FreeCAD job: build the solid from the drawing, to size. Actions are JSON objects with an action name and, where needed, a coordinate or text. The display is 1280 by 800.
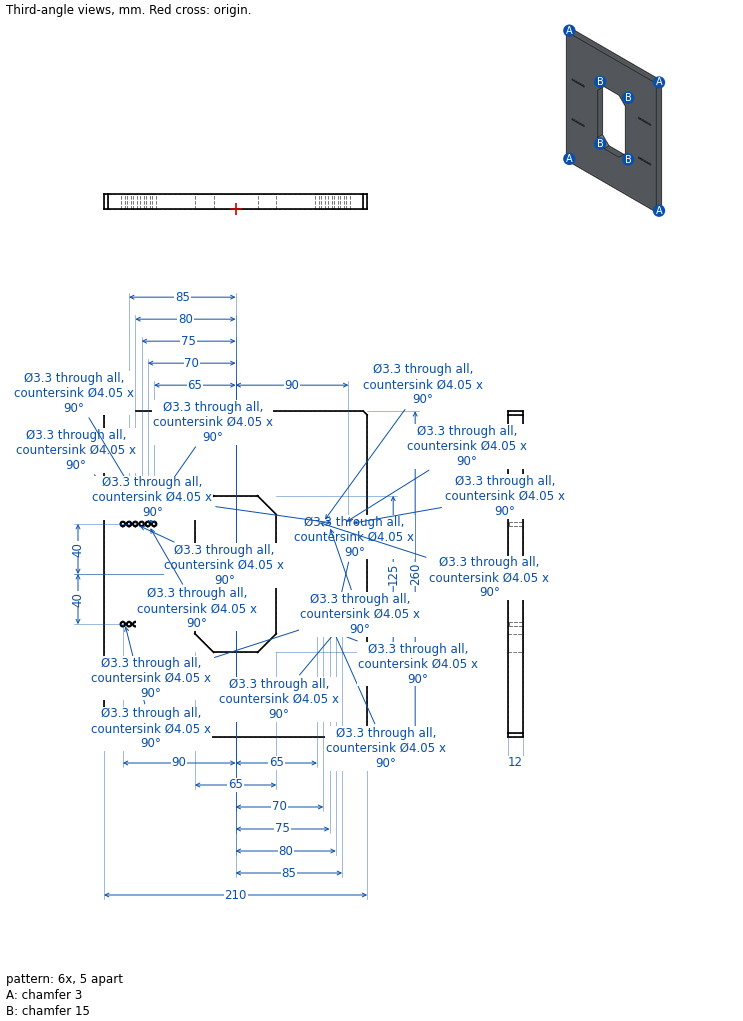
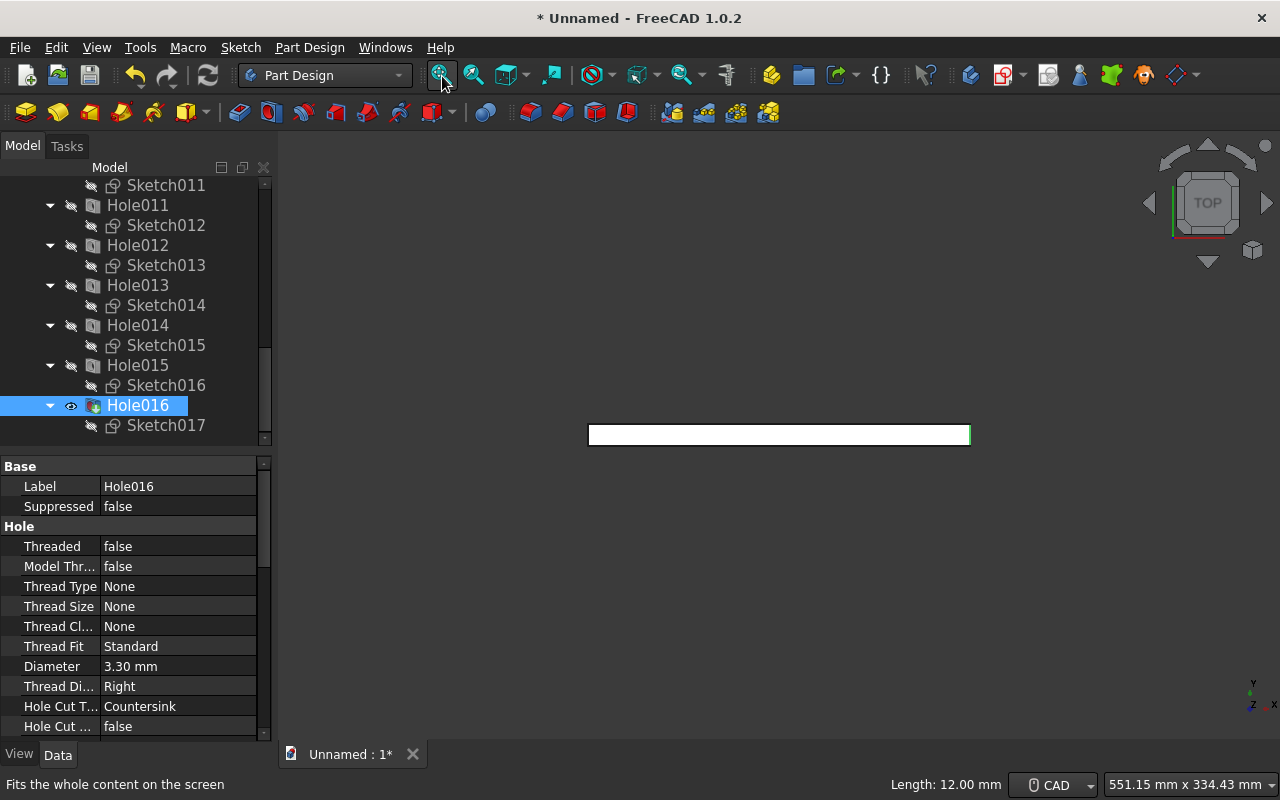
{"action": "left_click", "coordinate": [442, 76]}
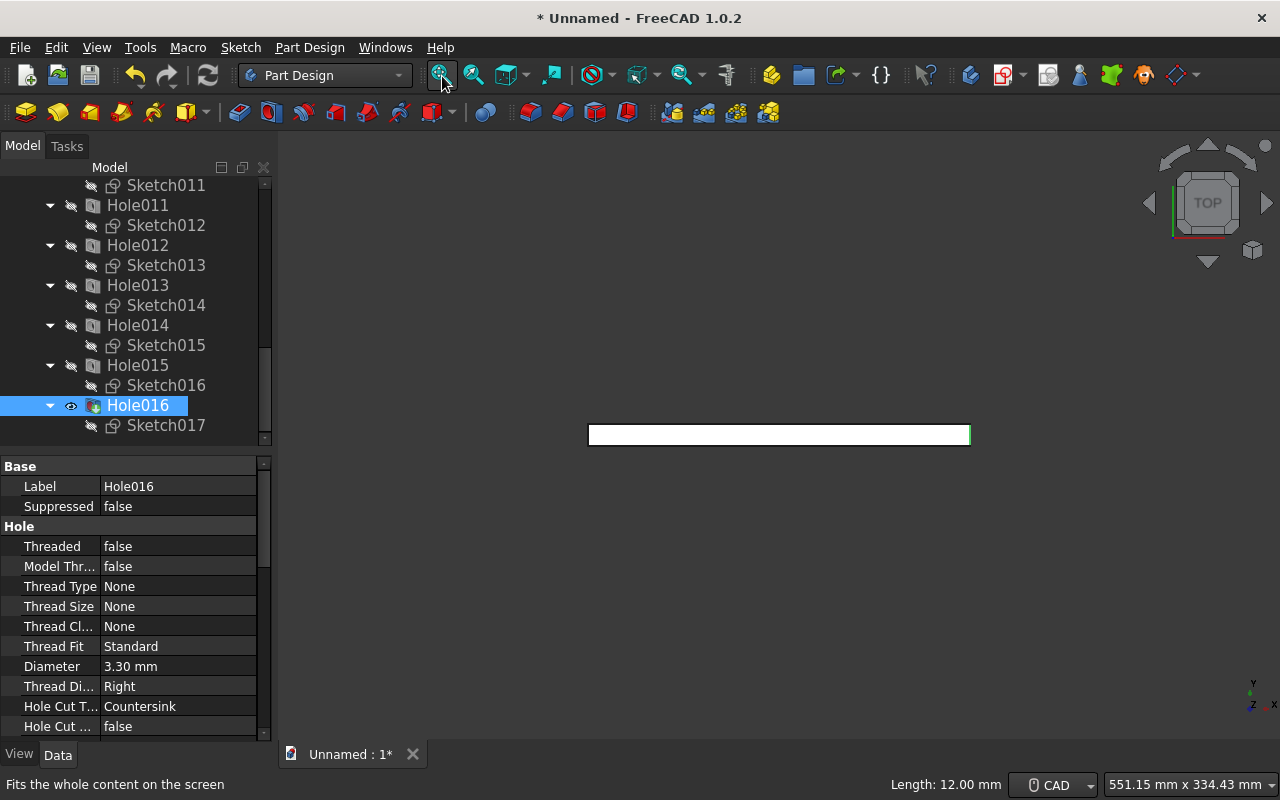
{"action": "left_click", "coordinate": [588, 434], "text": "ctrl"}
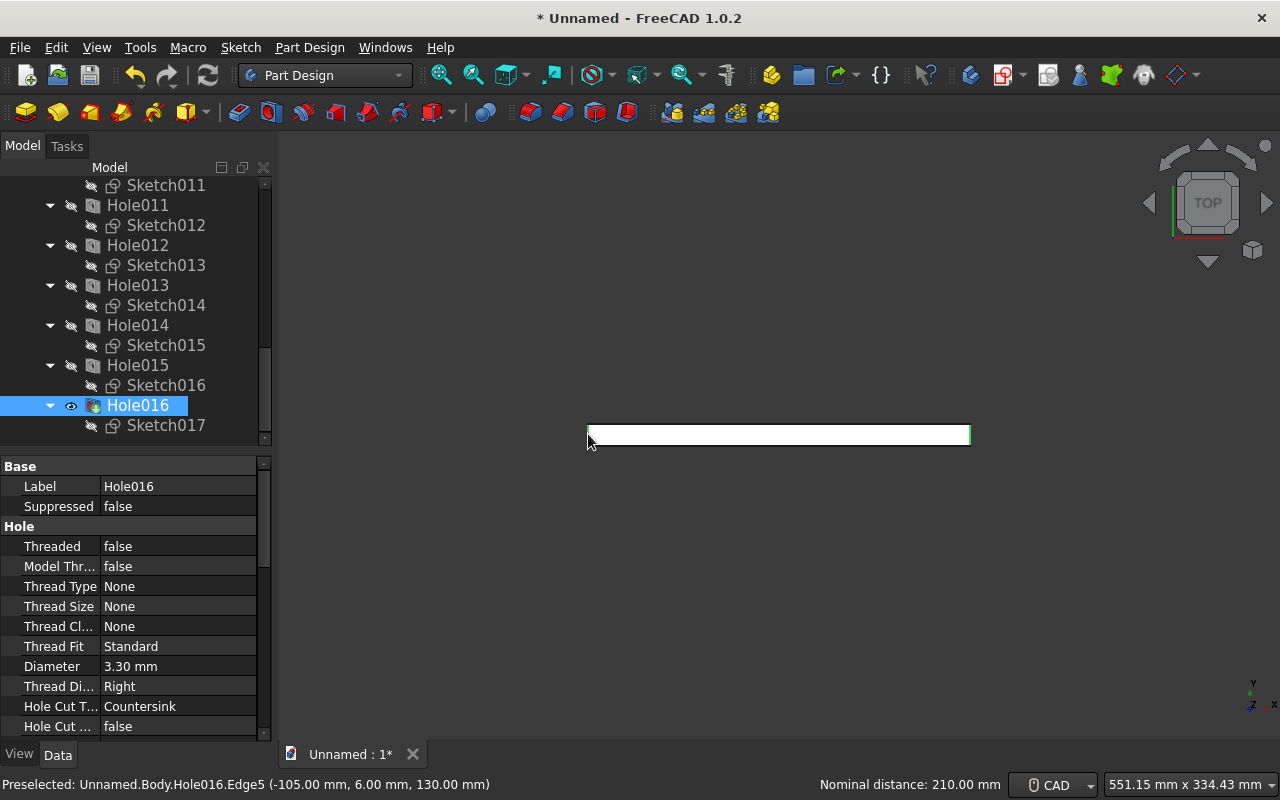
{"action": "scroll", "coordinate": [588, 434], "scroll_direction": "up", "scroll_amount": 4}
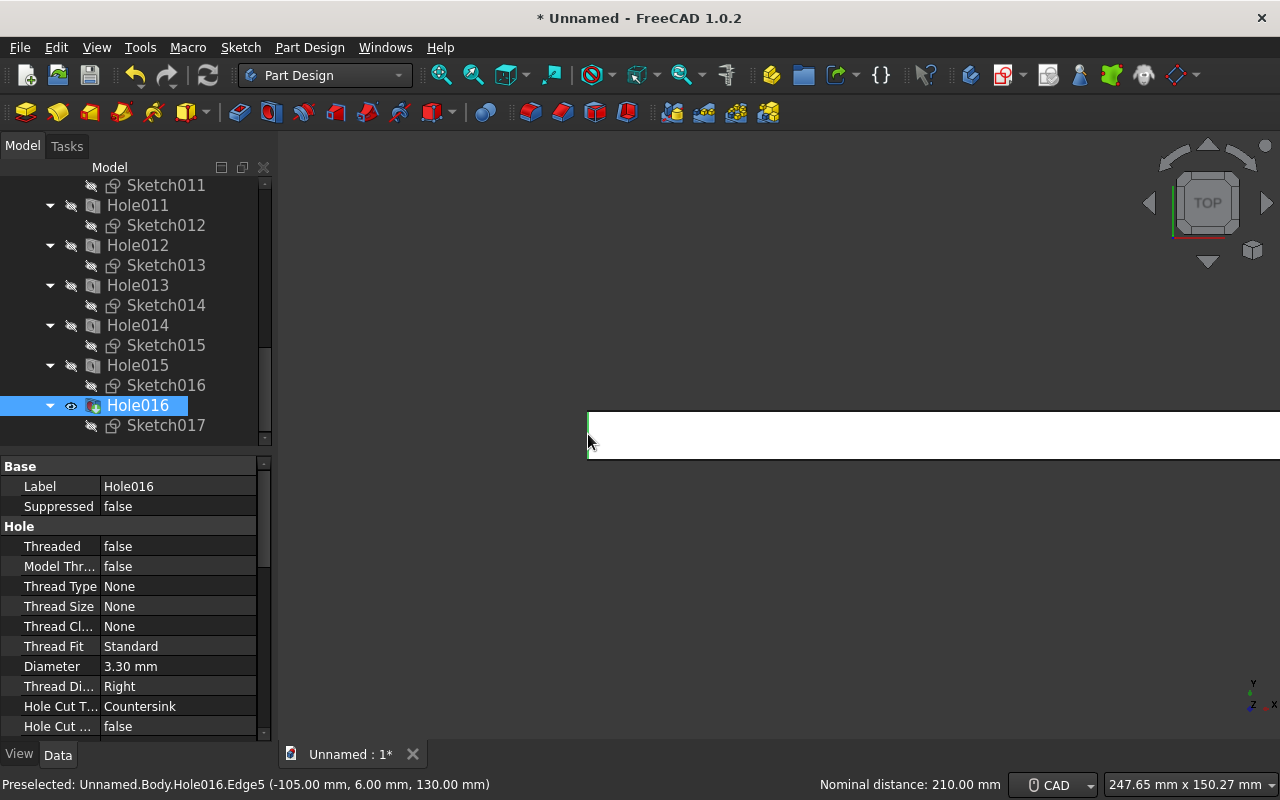
{"action": "left_click", "coordinate": [442, 76]}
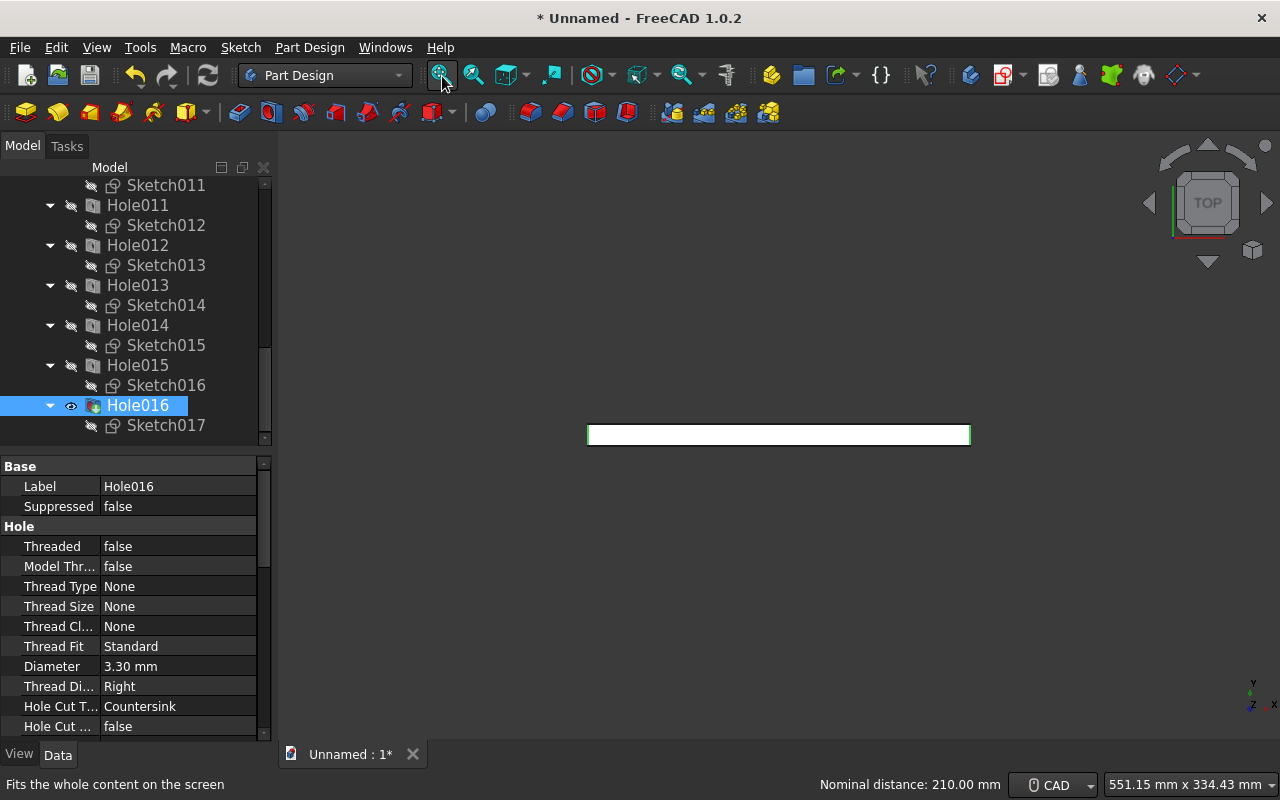
{"action": "key", "text": "1"}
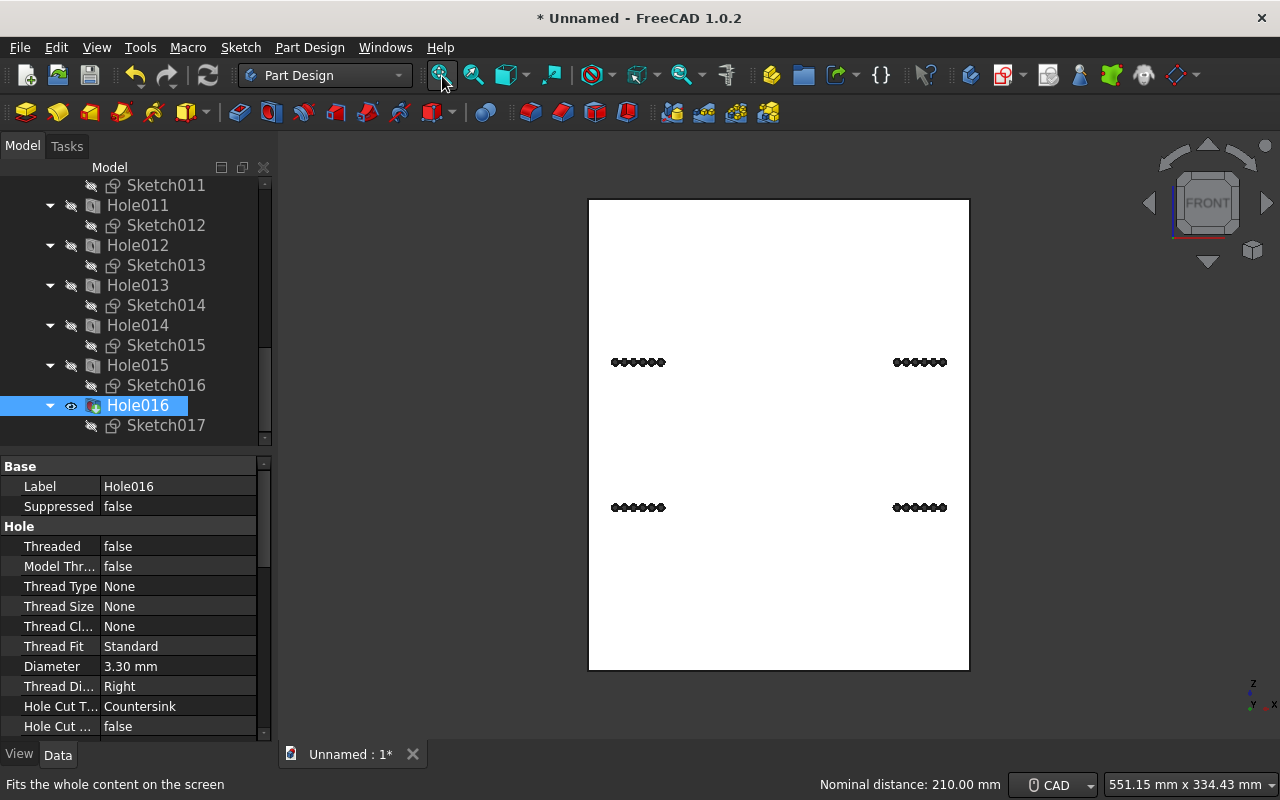
{"action": "scroll", "coordinate": [588, 670], "scroll_direction": "up", "scroll_amount": 4}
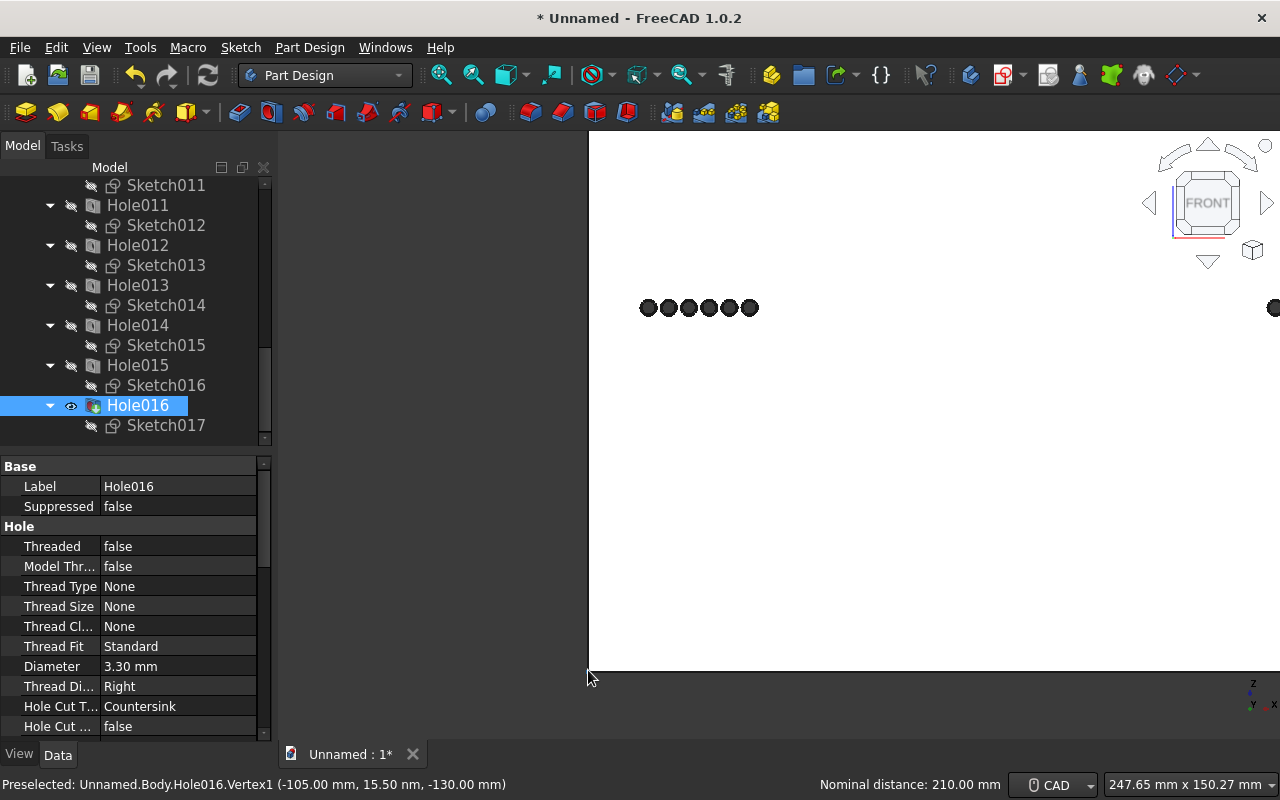
{"action": "left_click", "coordinate": [442, 76]}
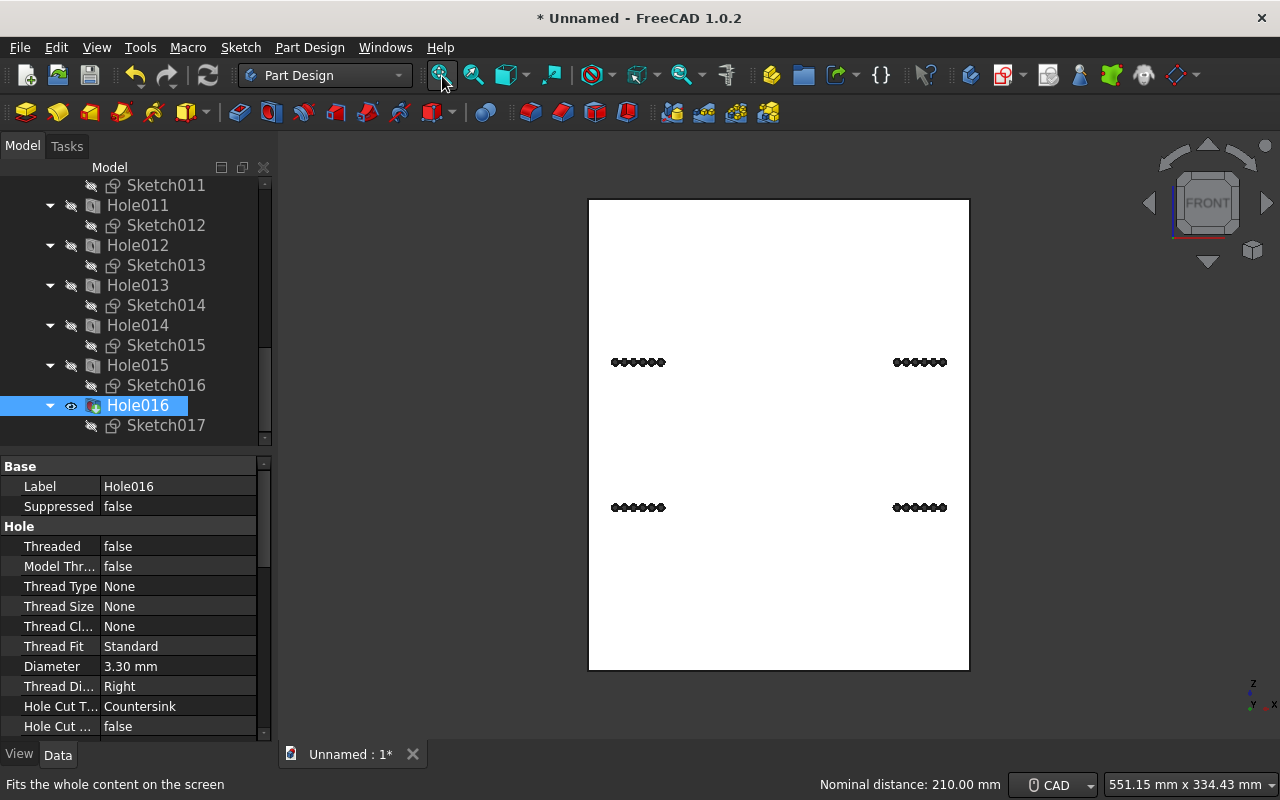
{"action": "key", "text": "3"}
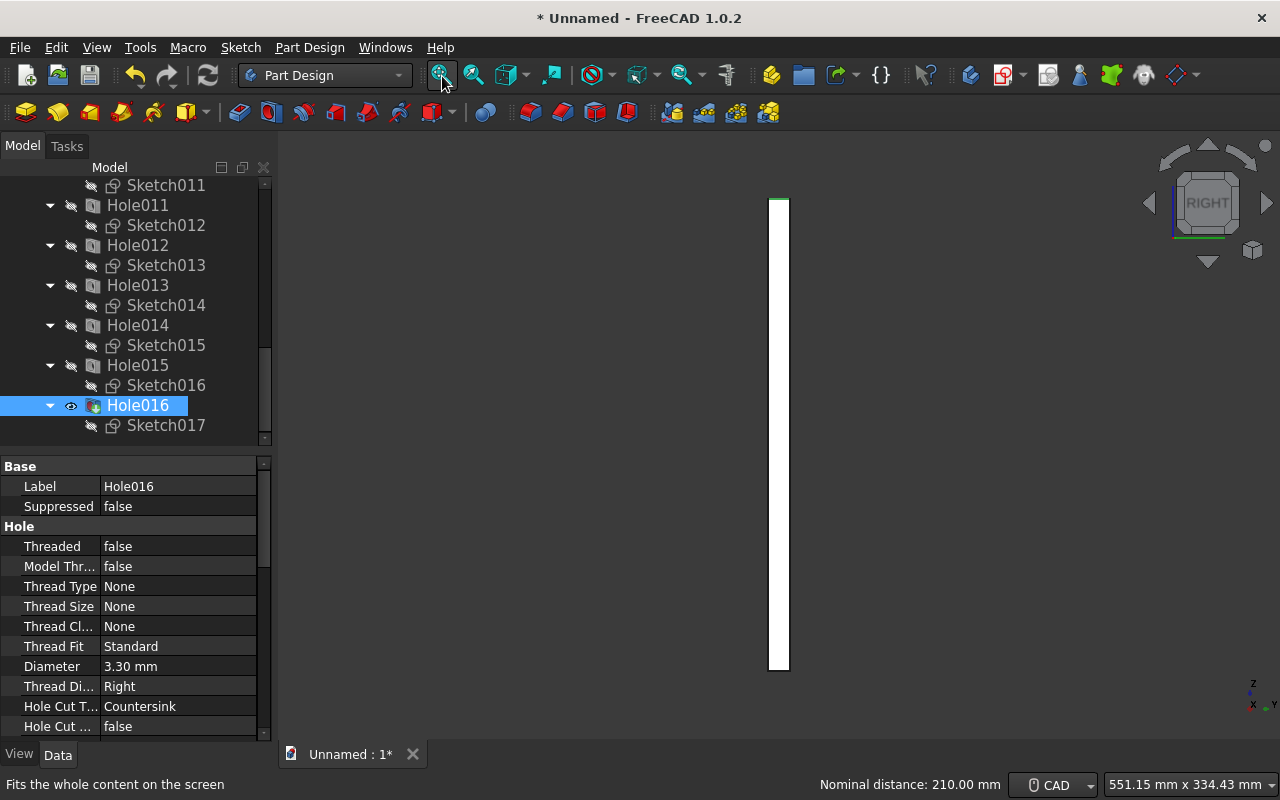
{"action": "left_click", "coordinate": [779, 670], "text": "ctrl"}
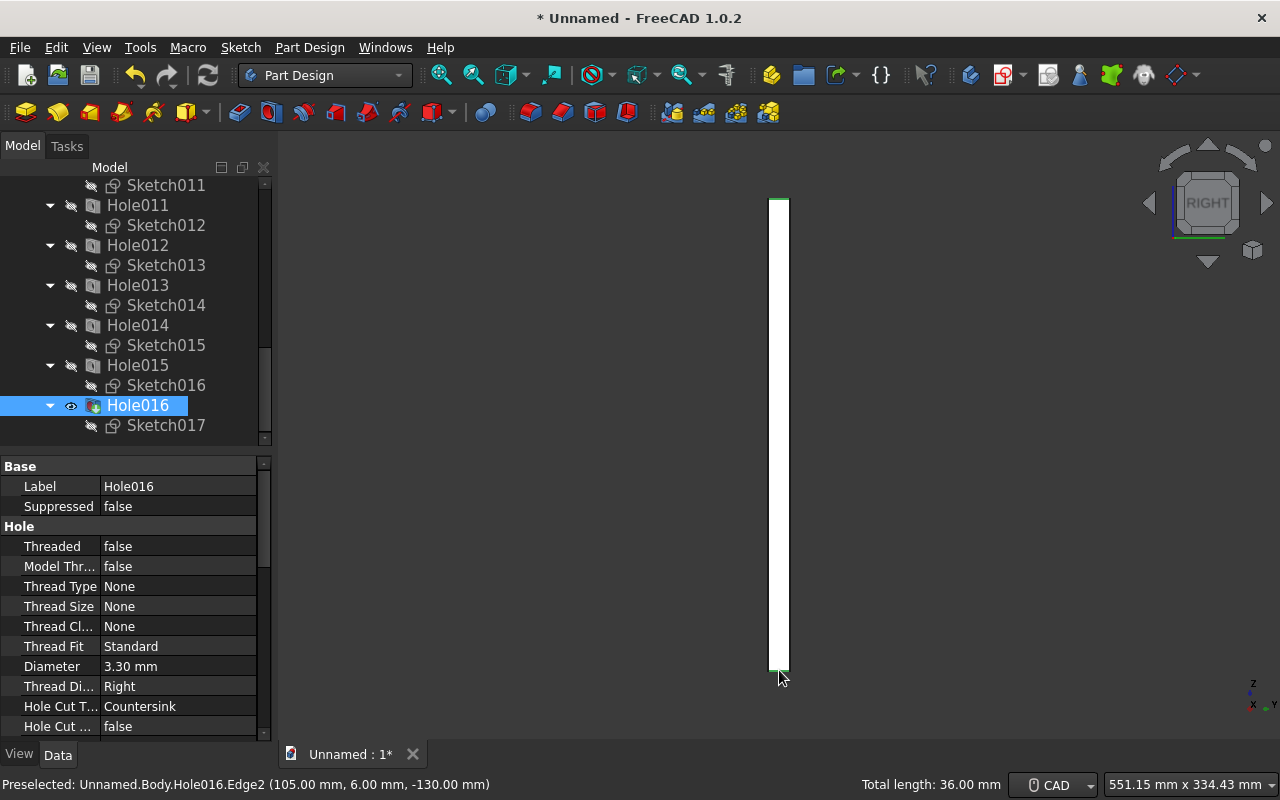
{"action": "scroll", "coordinate": [779, 670], "scroll_direction": "up", "scroll_amount": 4}